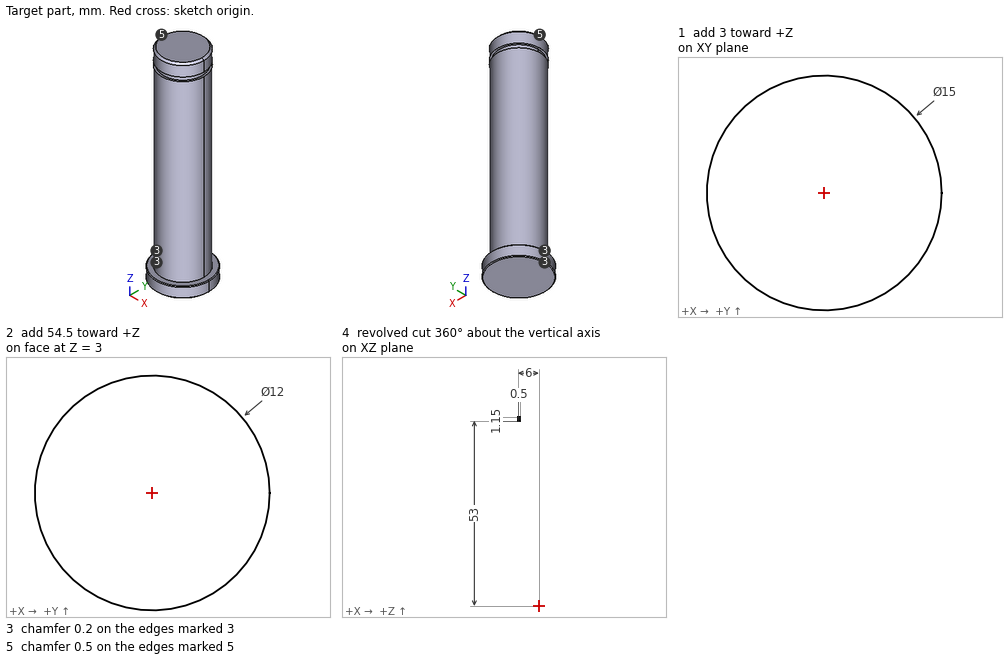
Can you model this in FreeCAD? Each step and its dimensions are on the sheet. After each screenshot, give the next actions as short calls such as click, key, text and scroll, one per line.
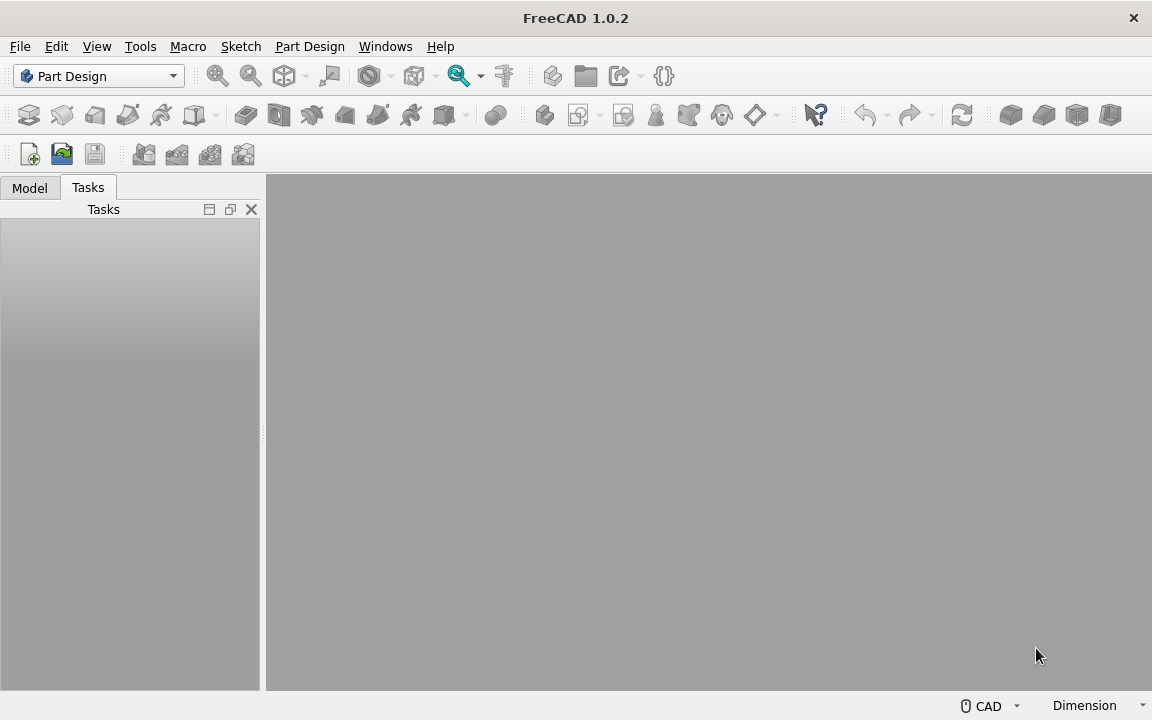
key(ctrl+n)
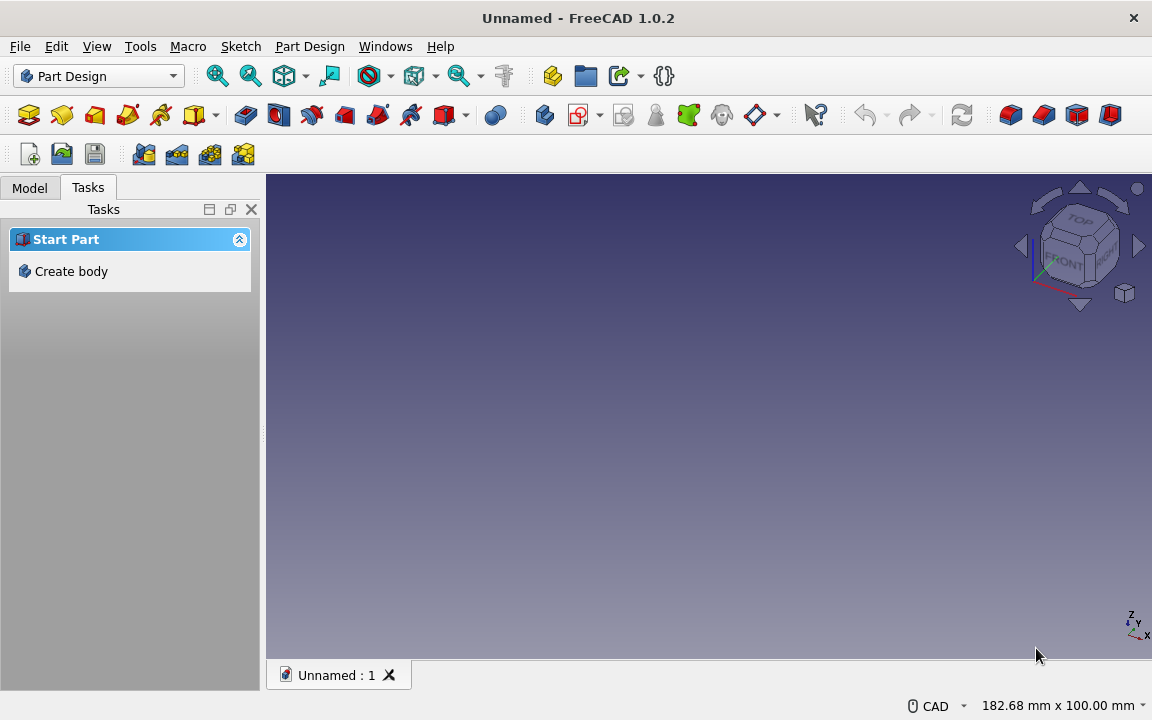
click(578, 116)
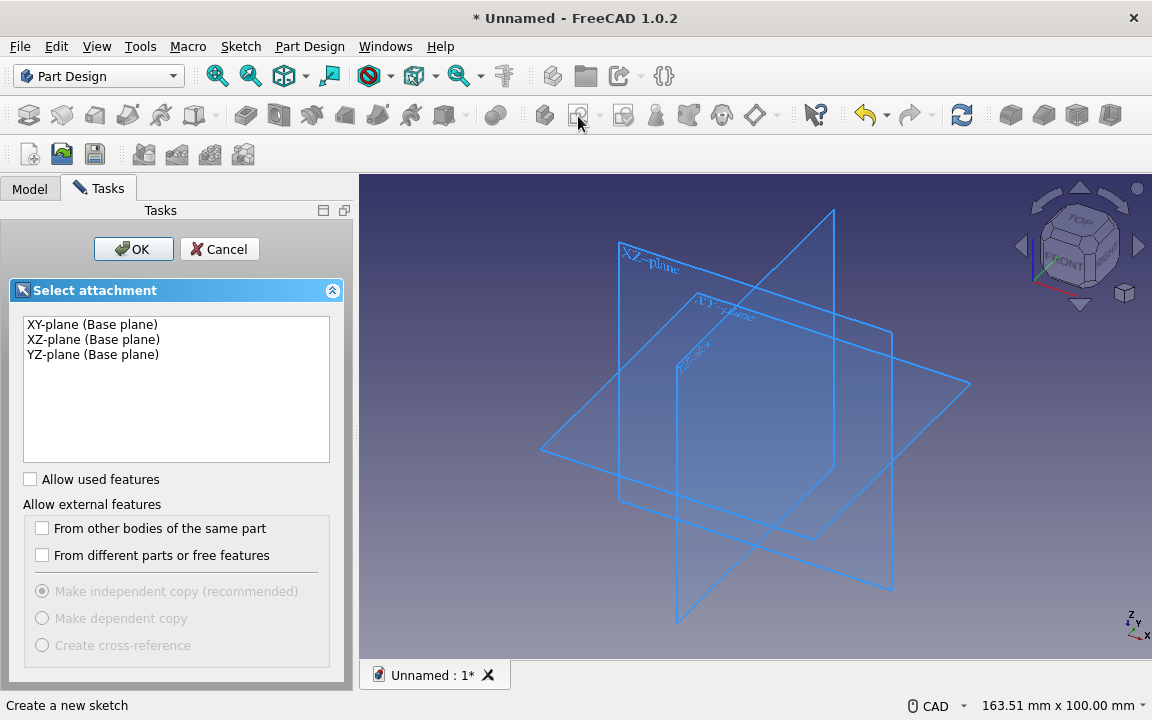
click(84, 324)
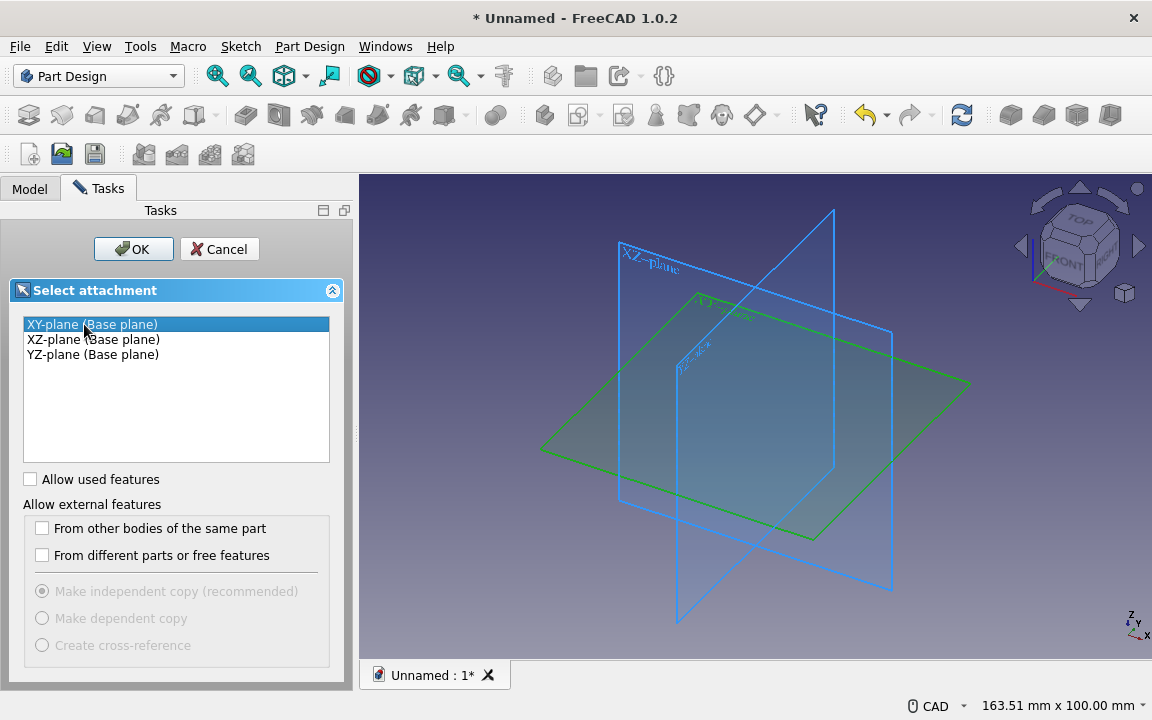
click(134, 249)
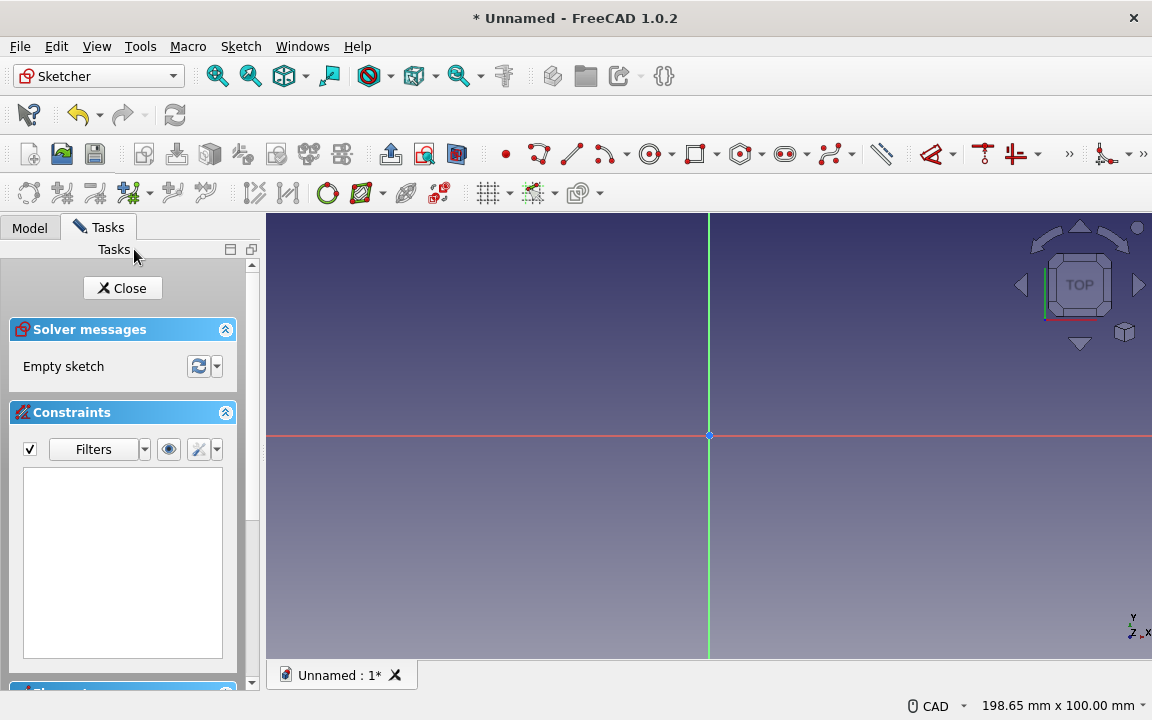
scroll(731, 436, up, 7)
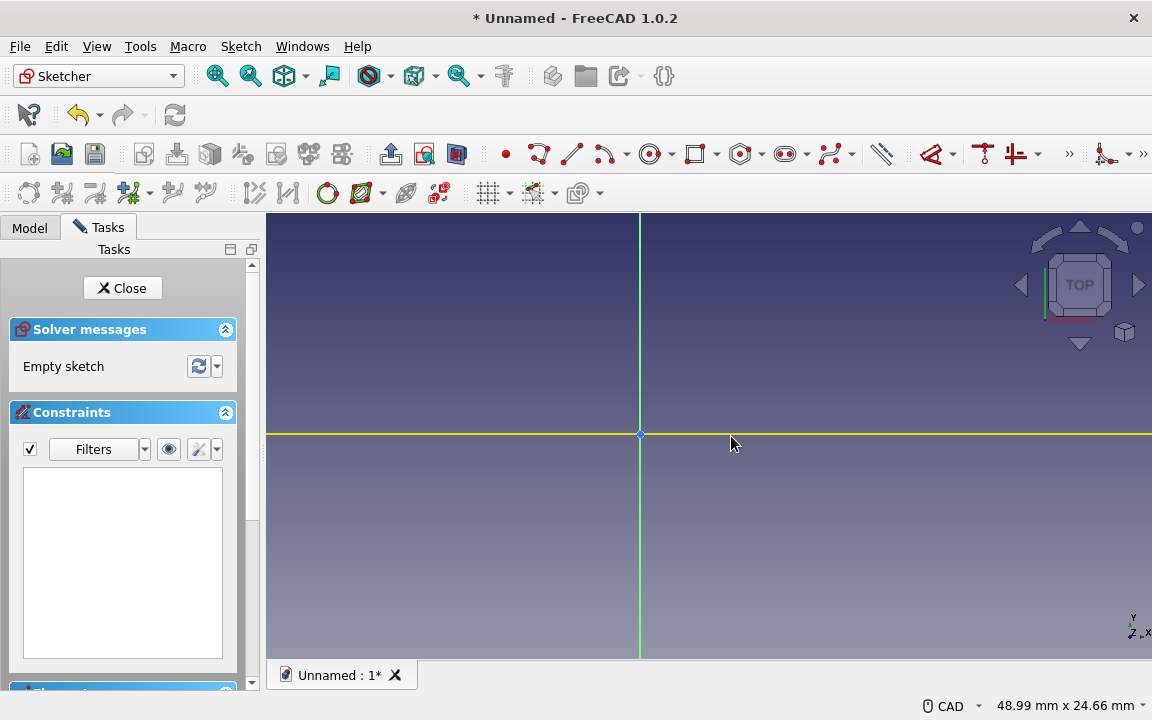
click(650, 154)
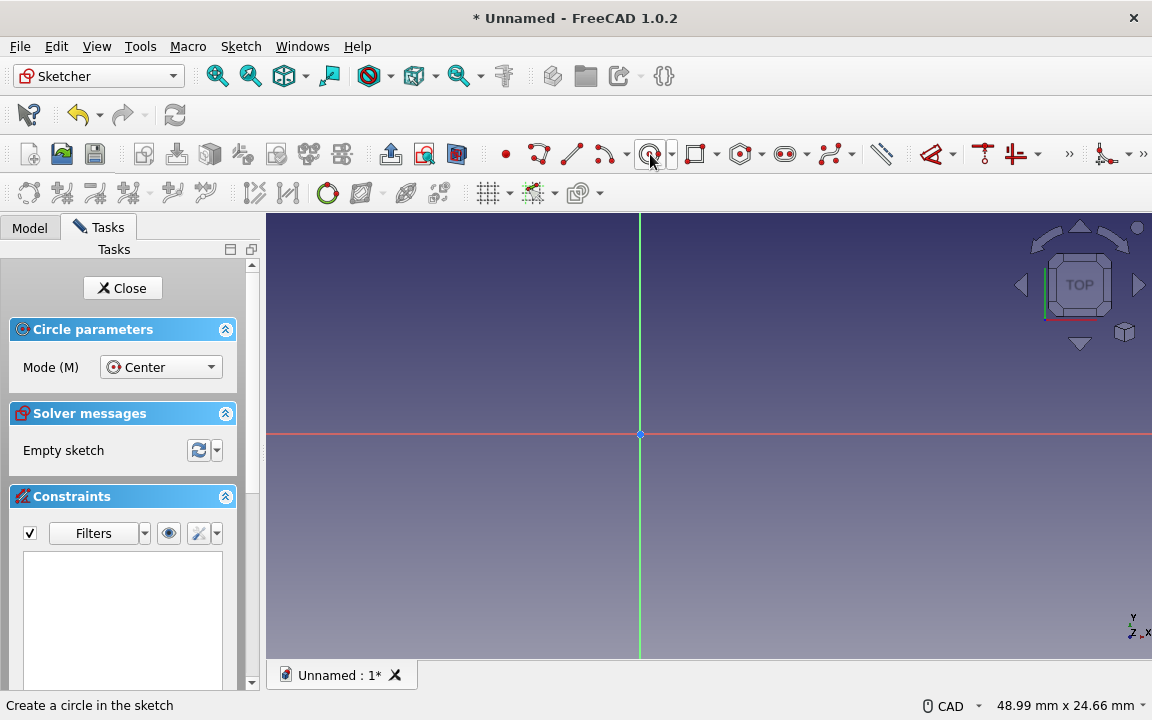
click(640, 434)
move(736, 339)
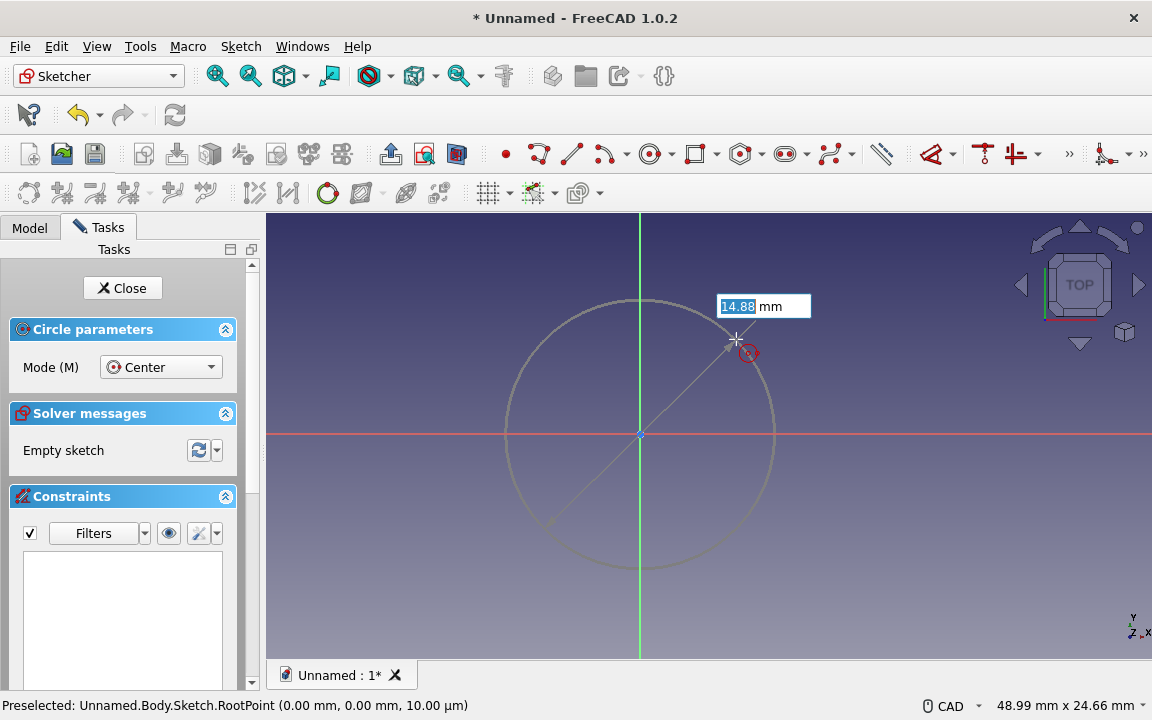
text(15)
key(Return)
key(Escape)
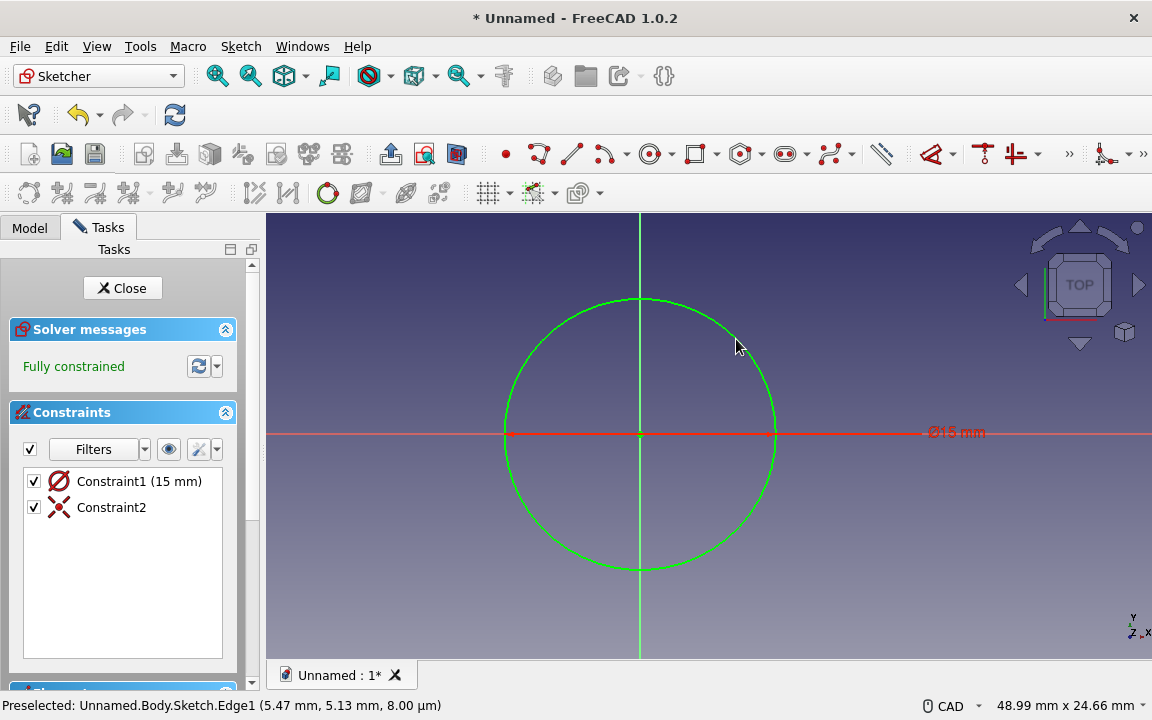
click(123, 288)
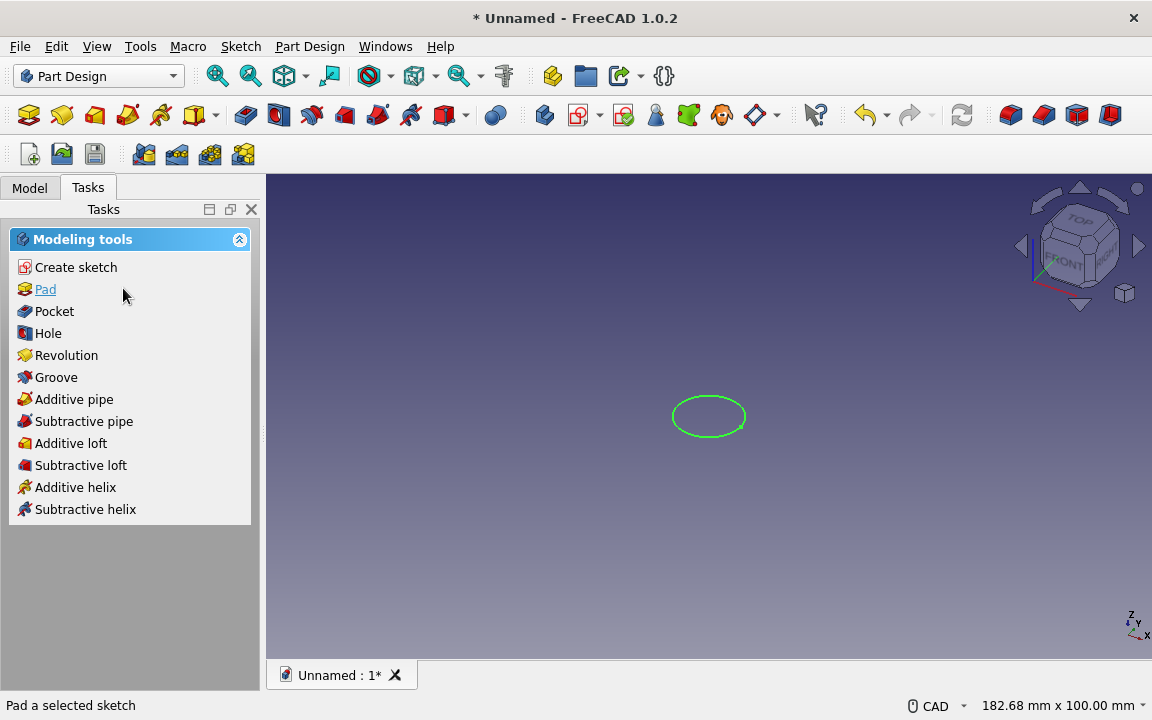
click(29, 116)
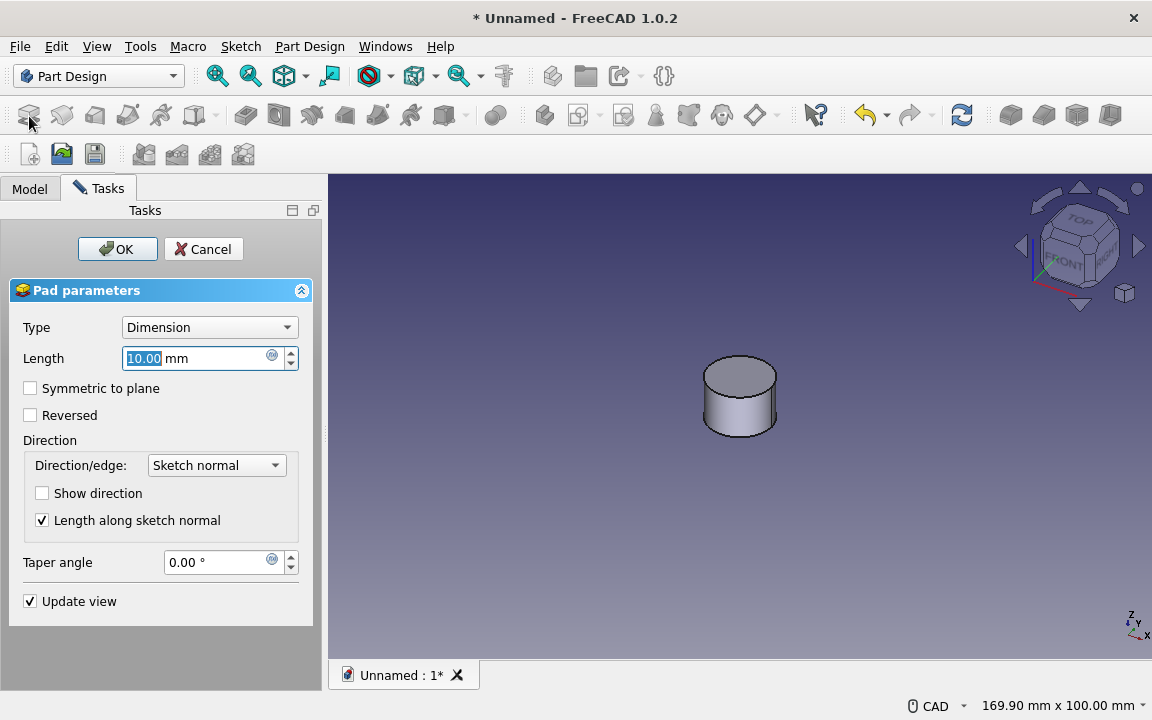
text(3)
key(Tab)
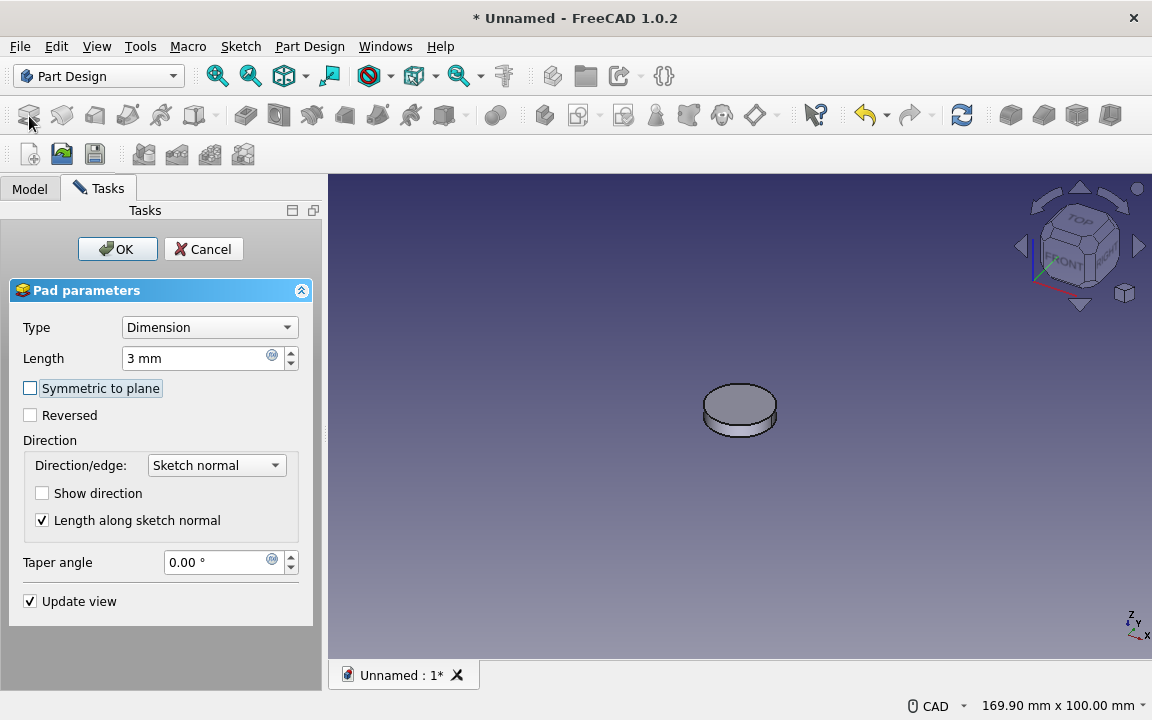
click(118, 249)